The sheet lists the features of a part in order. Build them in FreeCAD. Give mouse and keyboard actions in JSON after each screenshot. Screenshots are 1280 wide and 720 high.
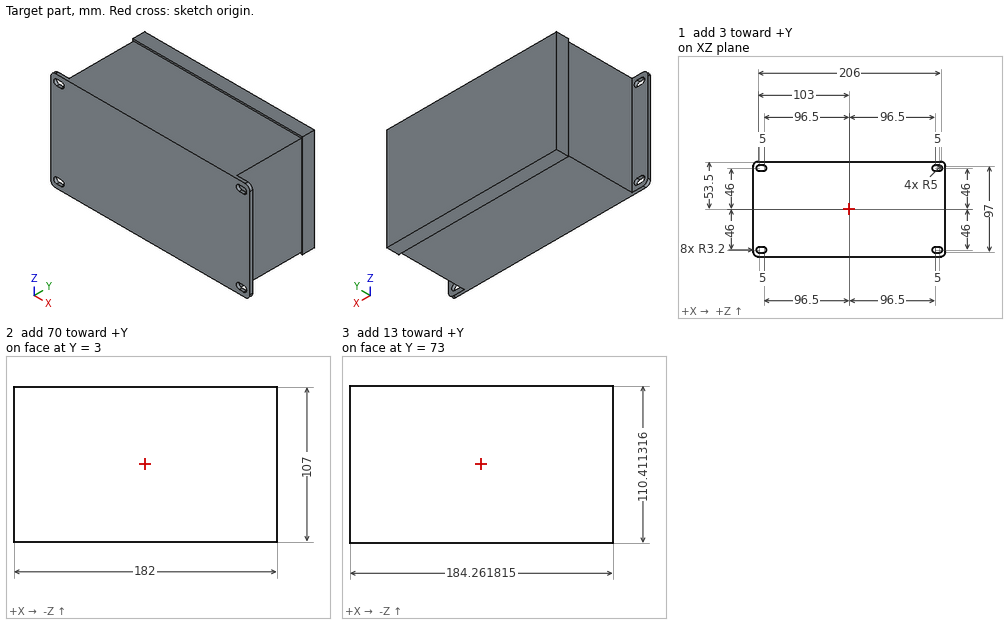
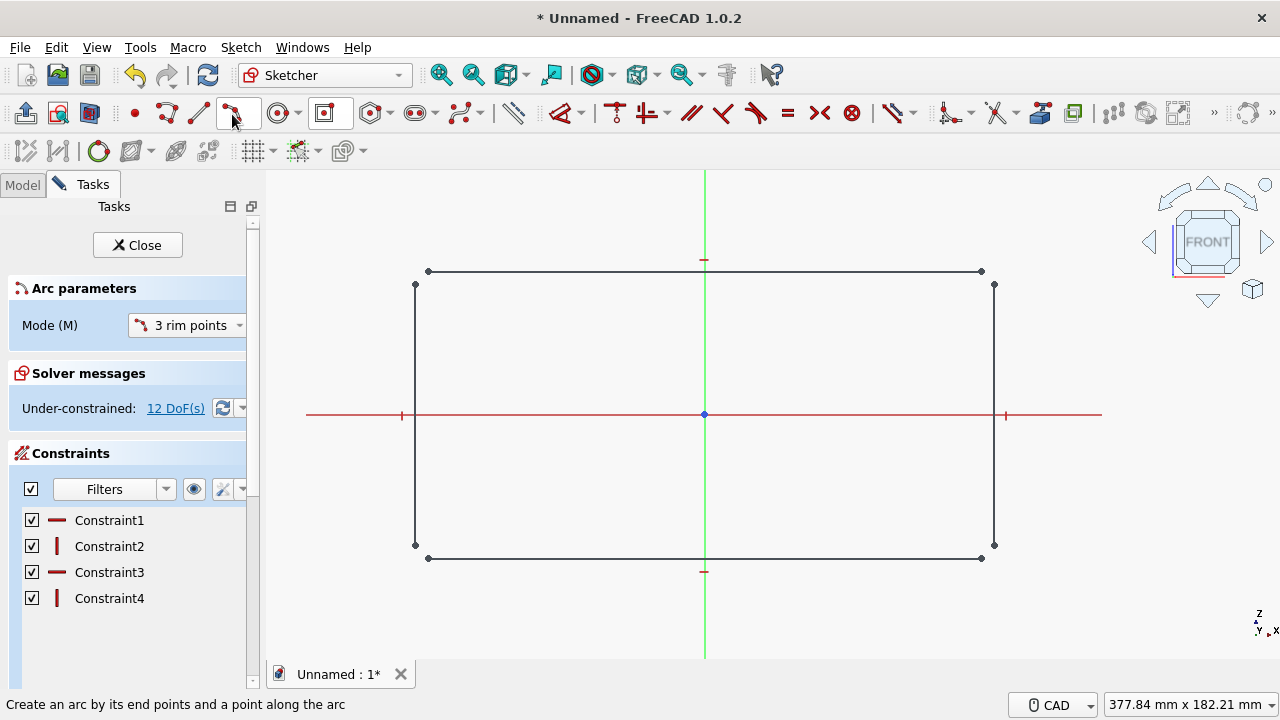
{"action": "left_click", "coordinate": [981, 272]}
{"action": "left_click", "coordinate": [994, 285]}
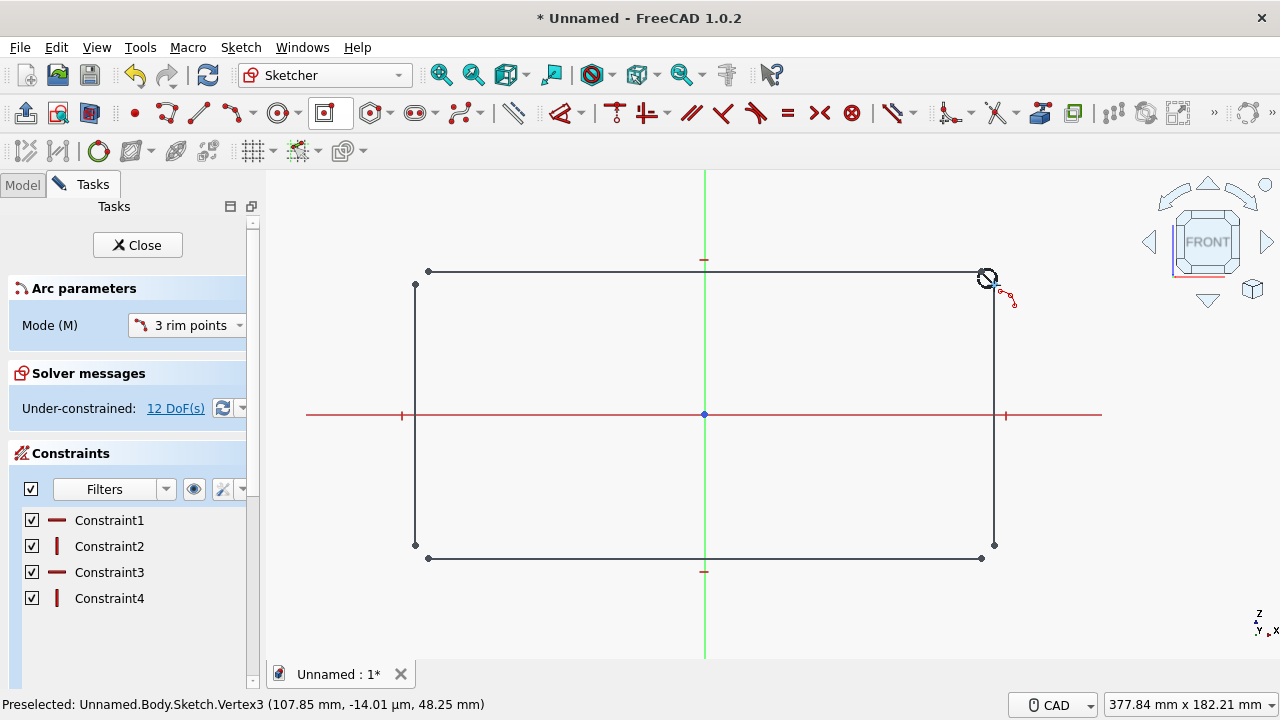
{"action": "scroll", "coordinate": [990, 275], "scroll_direction": "up", "scroll_amount": 7}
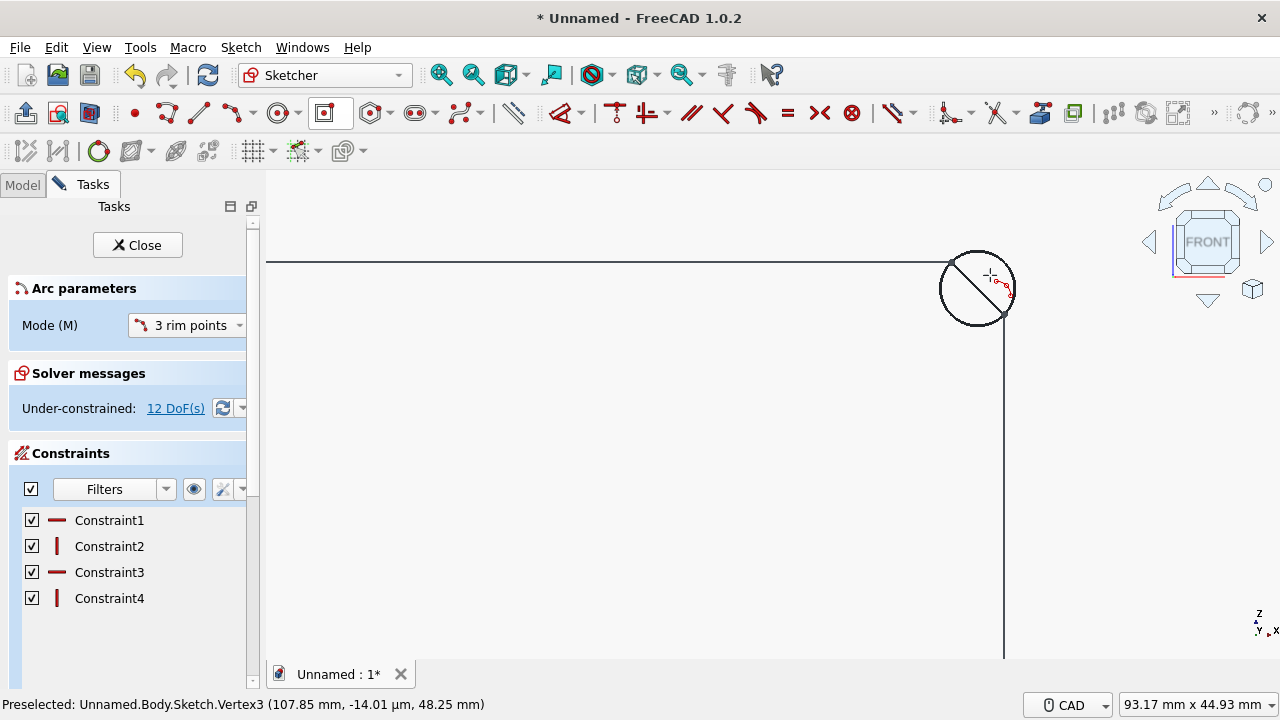
{"action": "left_click", "coordinate": [990, 274]}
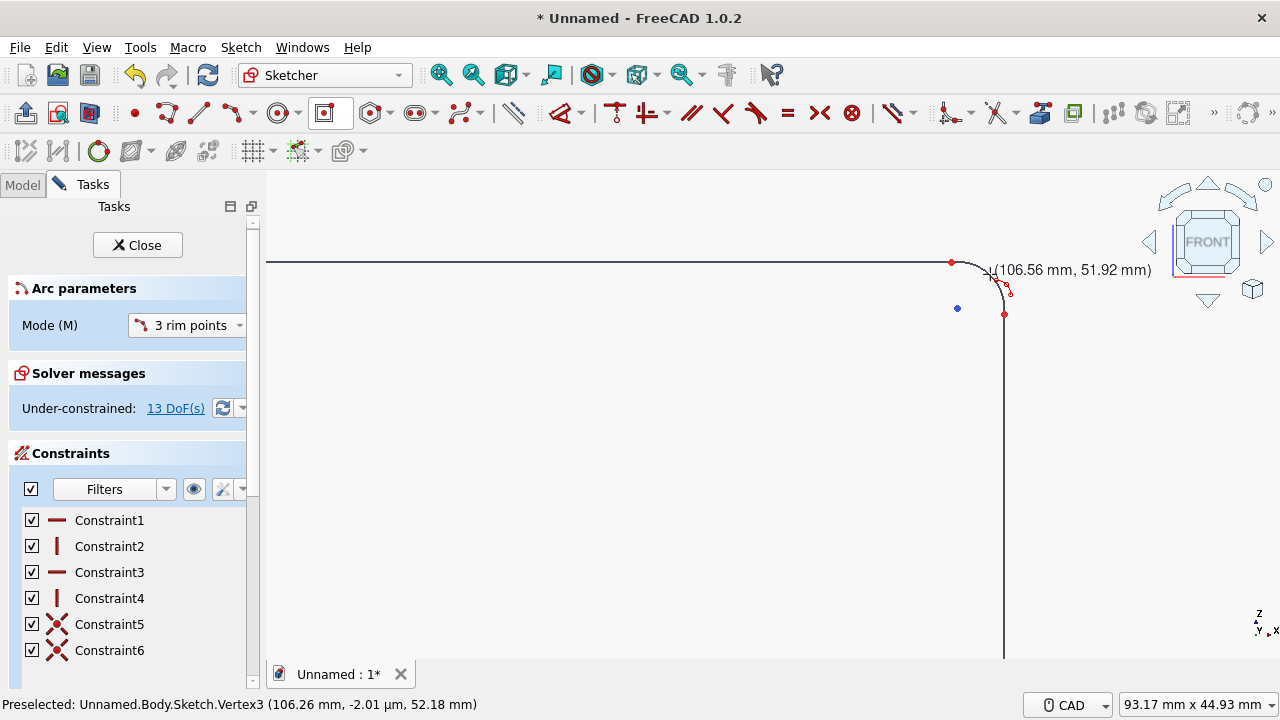
{"action": "scroll", "coordinate": [991, 275], "scroll_direction": "down", "scroll_amount": 7}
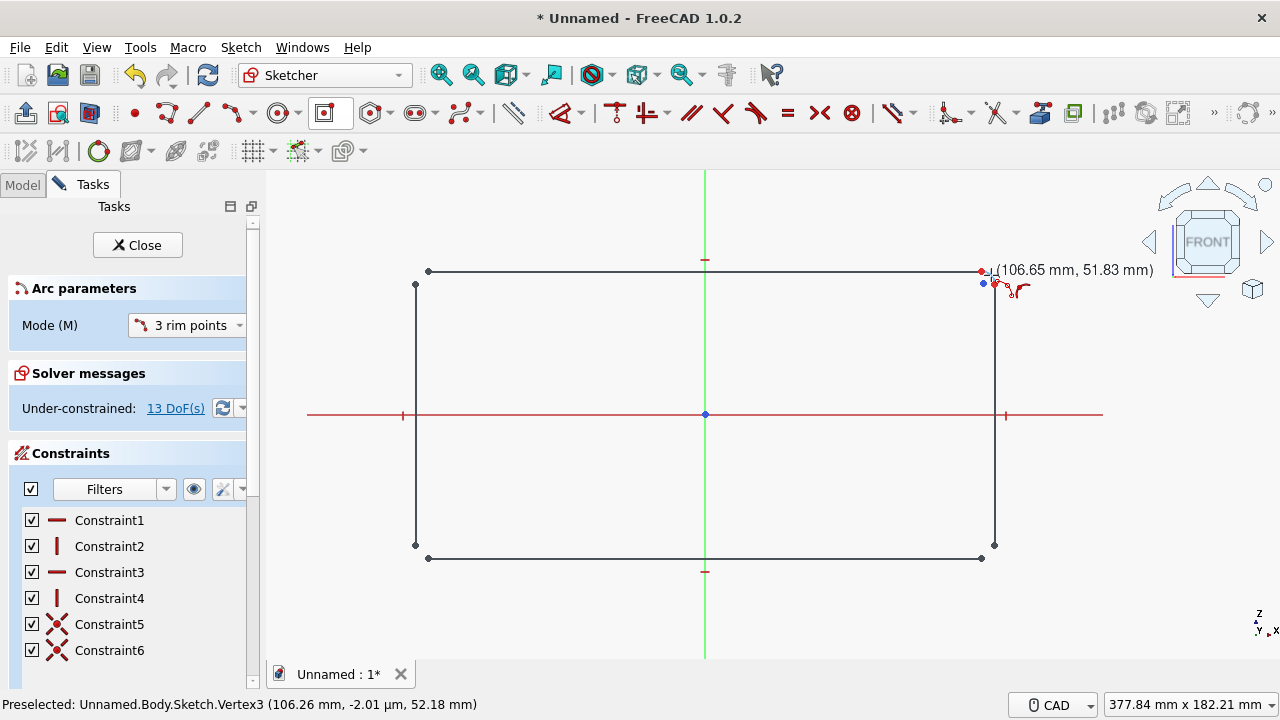
{"action": "left_click", "coordinate": [995, 546]}
{"action": "left_click", "coordinate": [982, 559]}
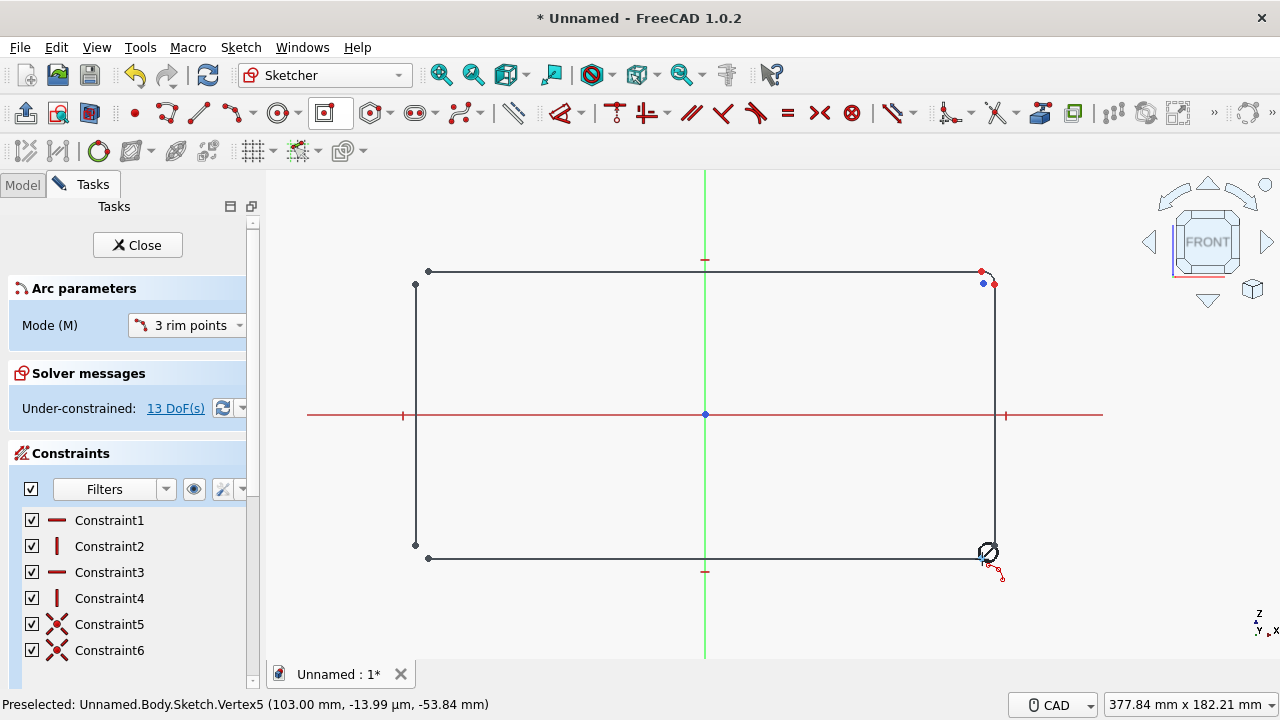
{"action": "scroll", "coordinate": [991, 554], "scroll_direction": "up", "scroll_amount": 7}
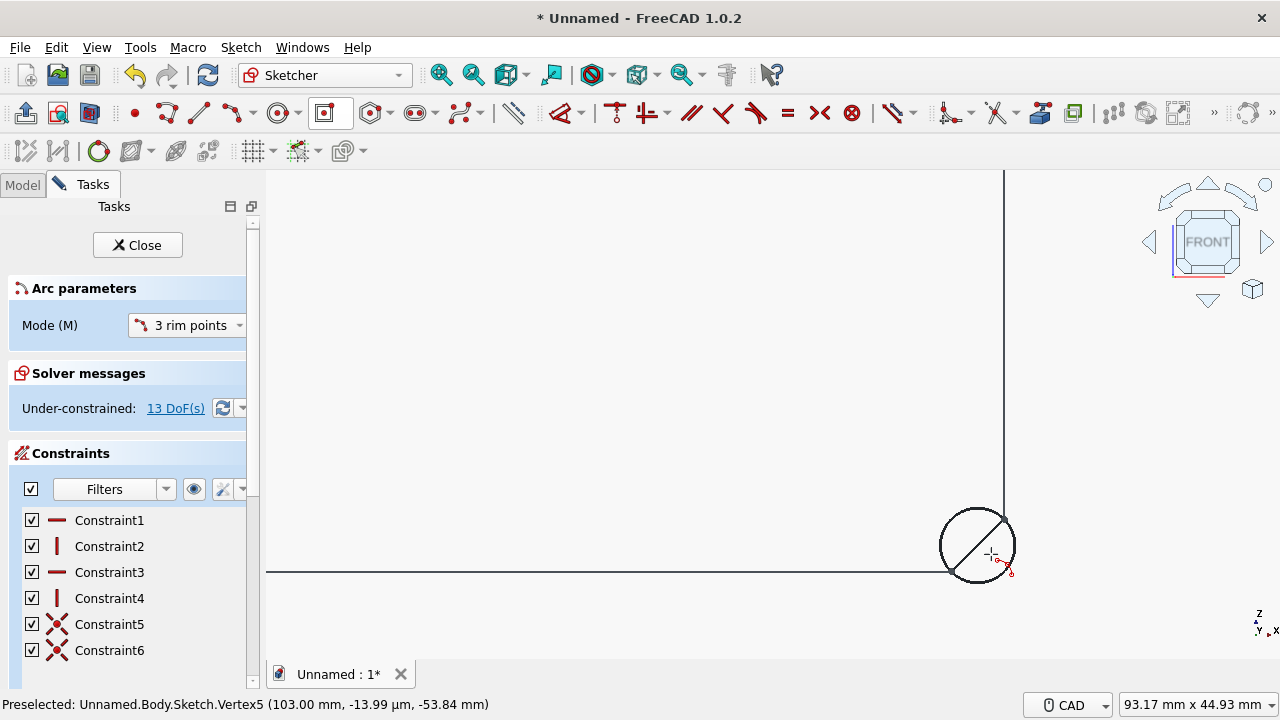
{"action": "left_click", "coordinate": [990, 552]}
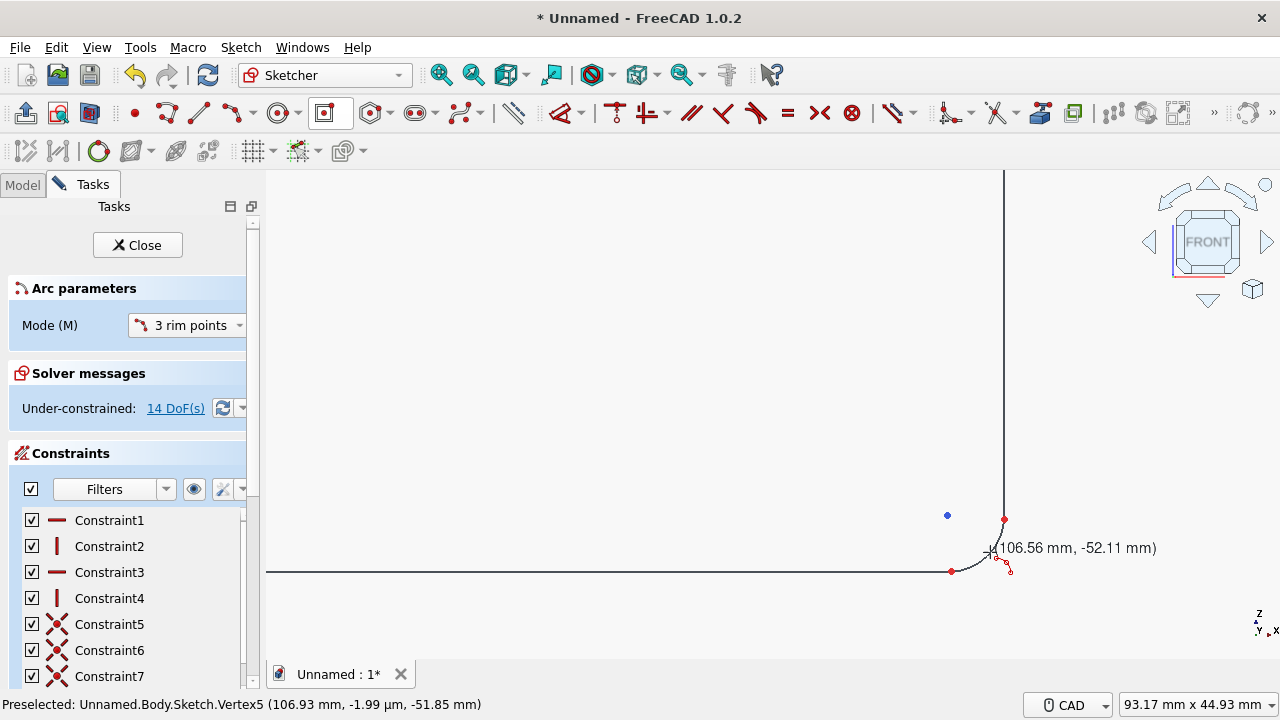
{"action": "scroll", "coordinate": [991, 555], "scroll_direction": "down", "scroll_amount": 7}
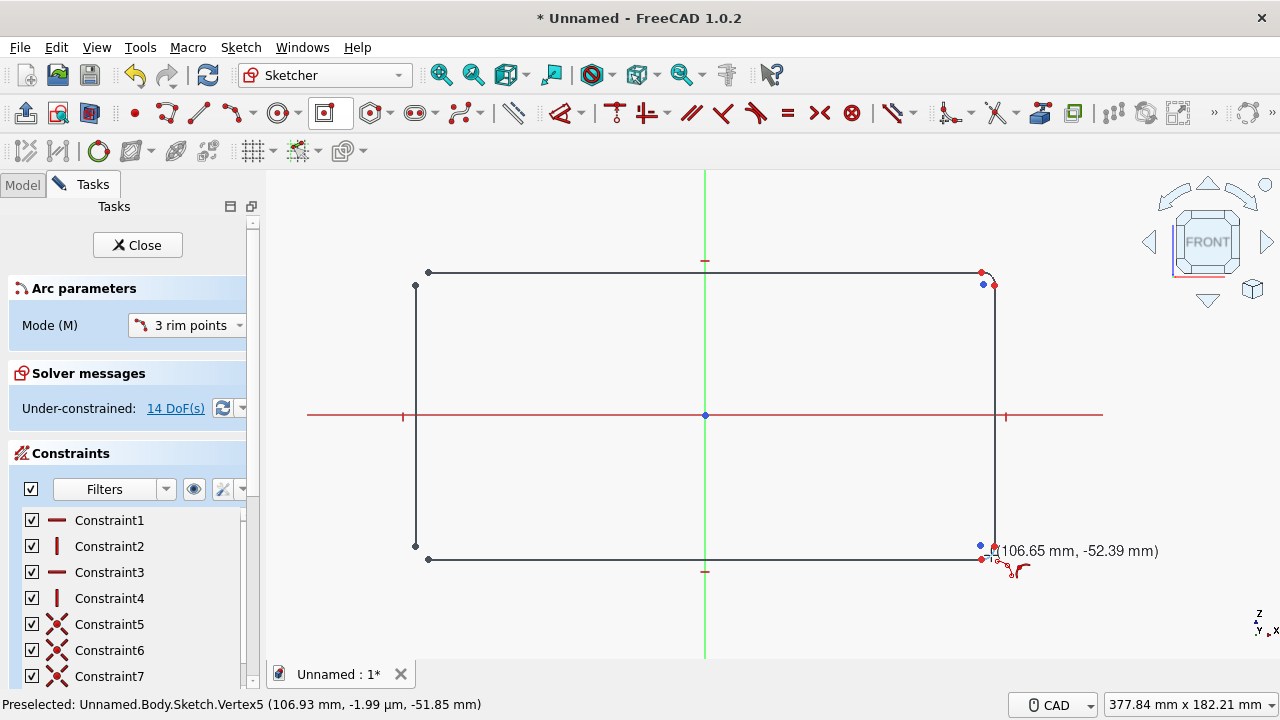
{"action": "left_click", "coordinate": [429, 560]}
{"action": "left_click", "coordinate": [416, 547]}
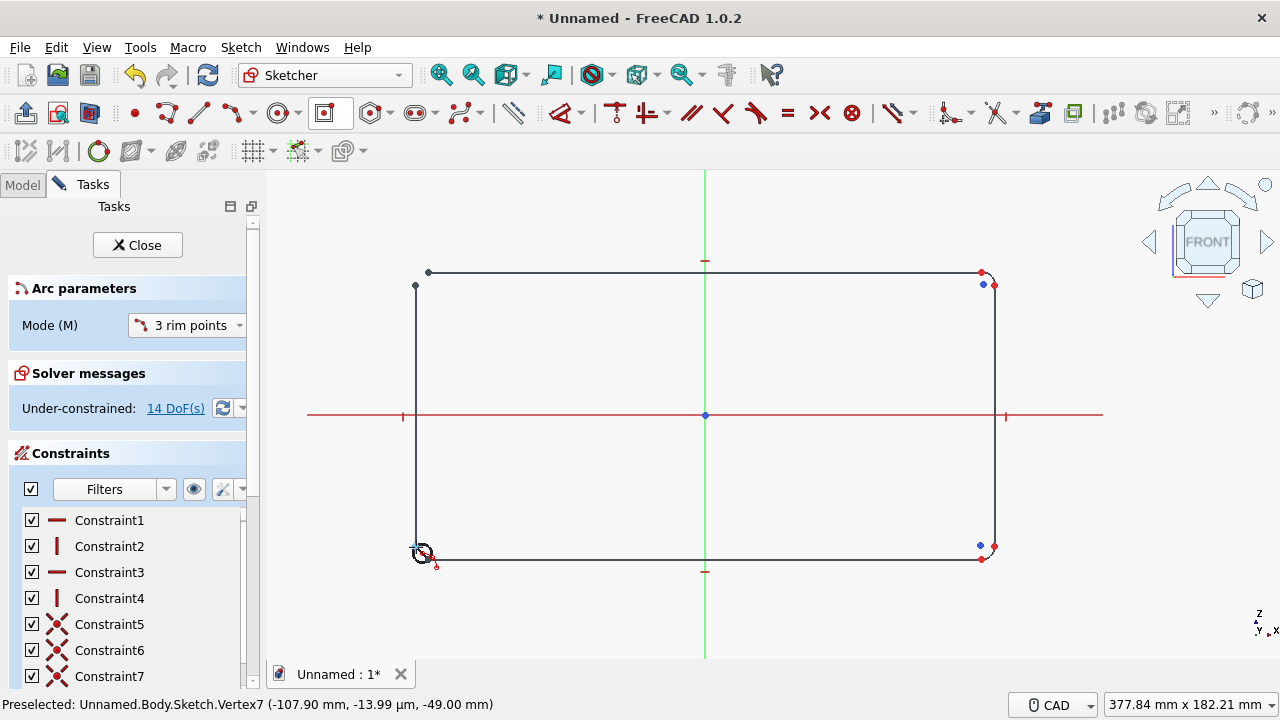
{"action": "scroll", "coordinate": [419, 555], "scroll_direction": "up", "scroll_amount": 7}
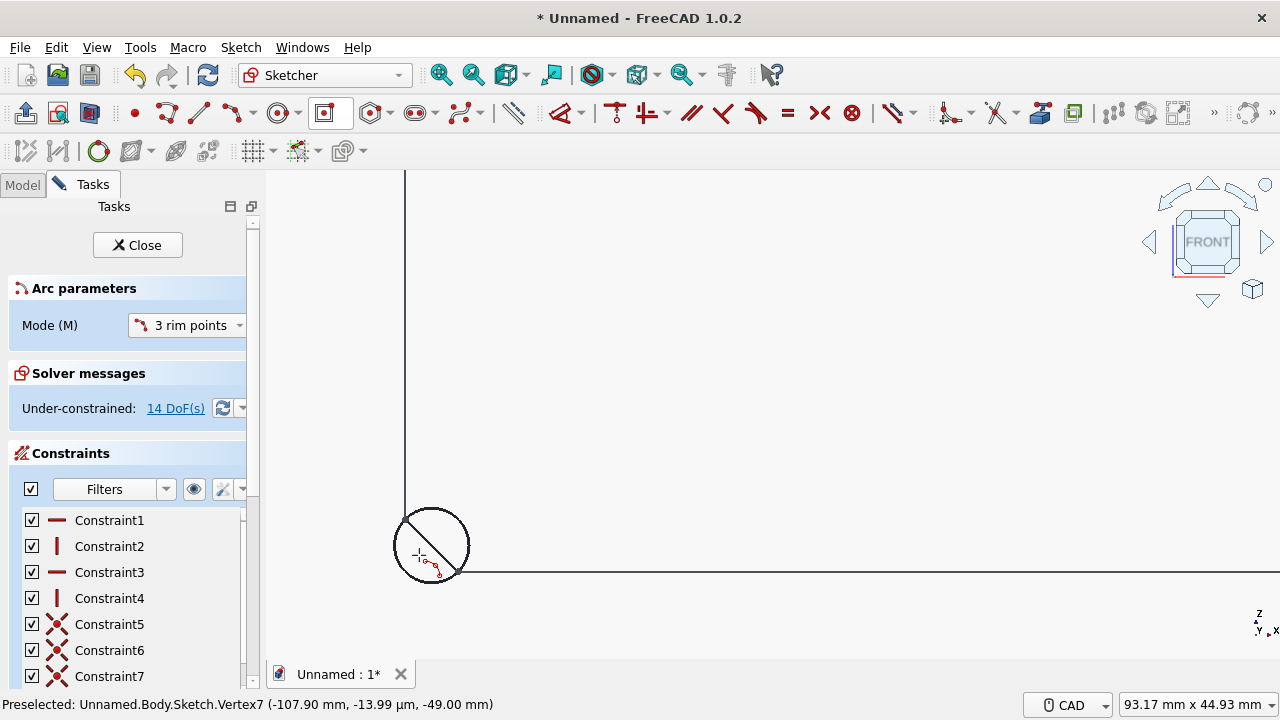
{"action": "left_click", "coordinate": [420, 552]}